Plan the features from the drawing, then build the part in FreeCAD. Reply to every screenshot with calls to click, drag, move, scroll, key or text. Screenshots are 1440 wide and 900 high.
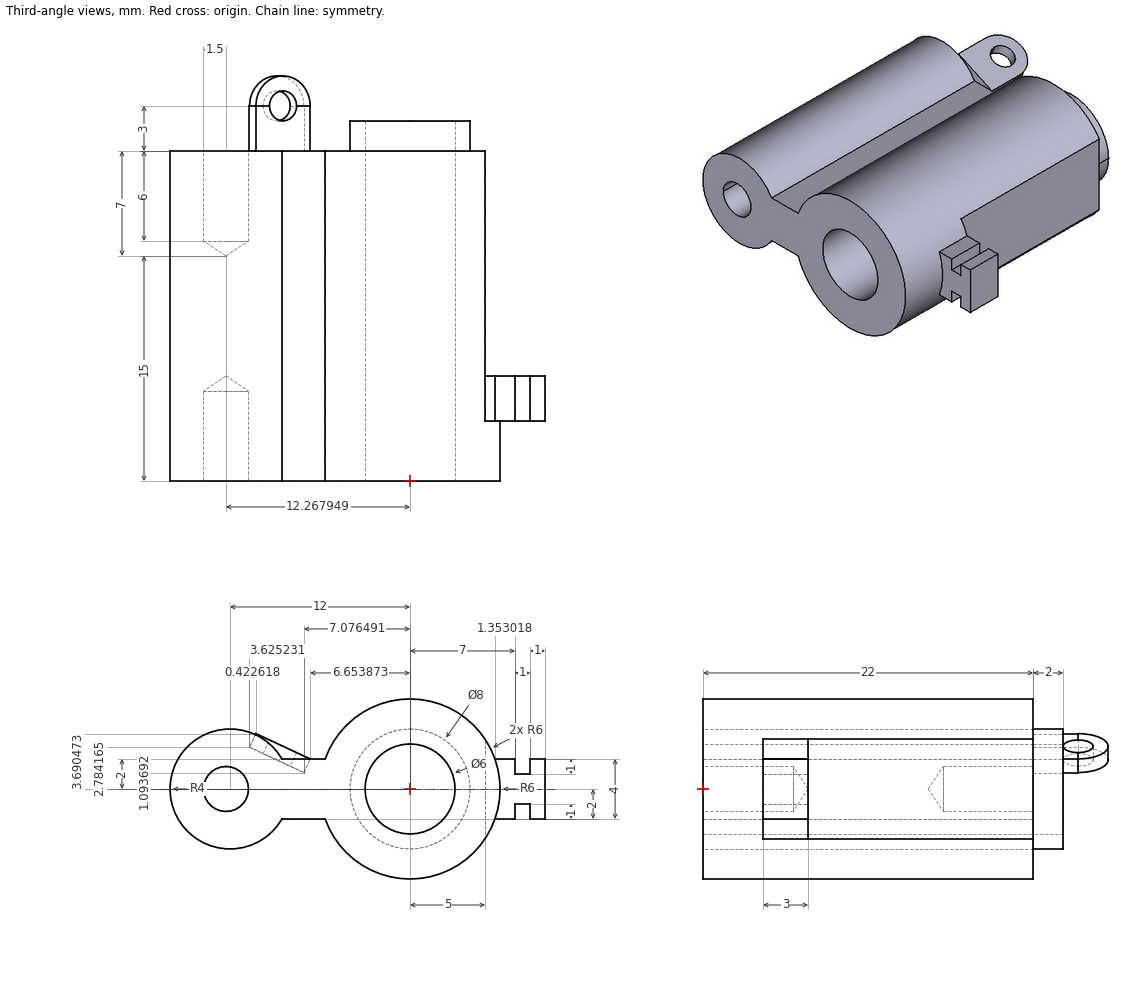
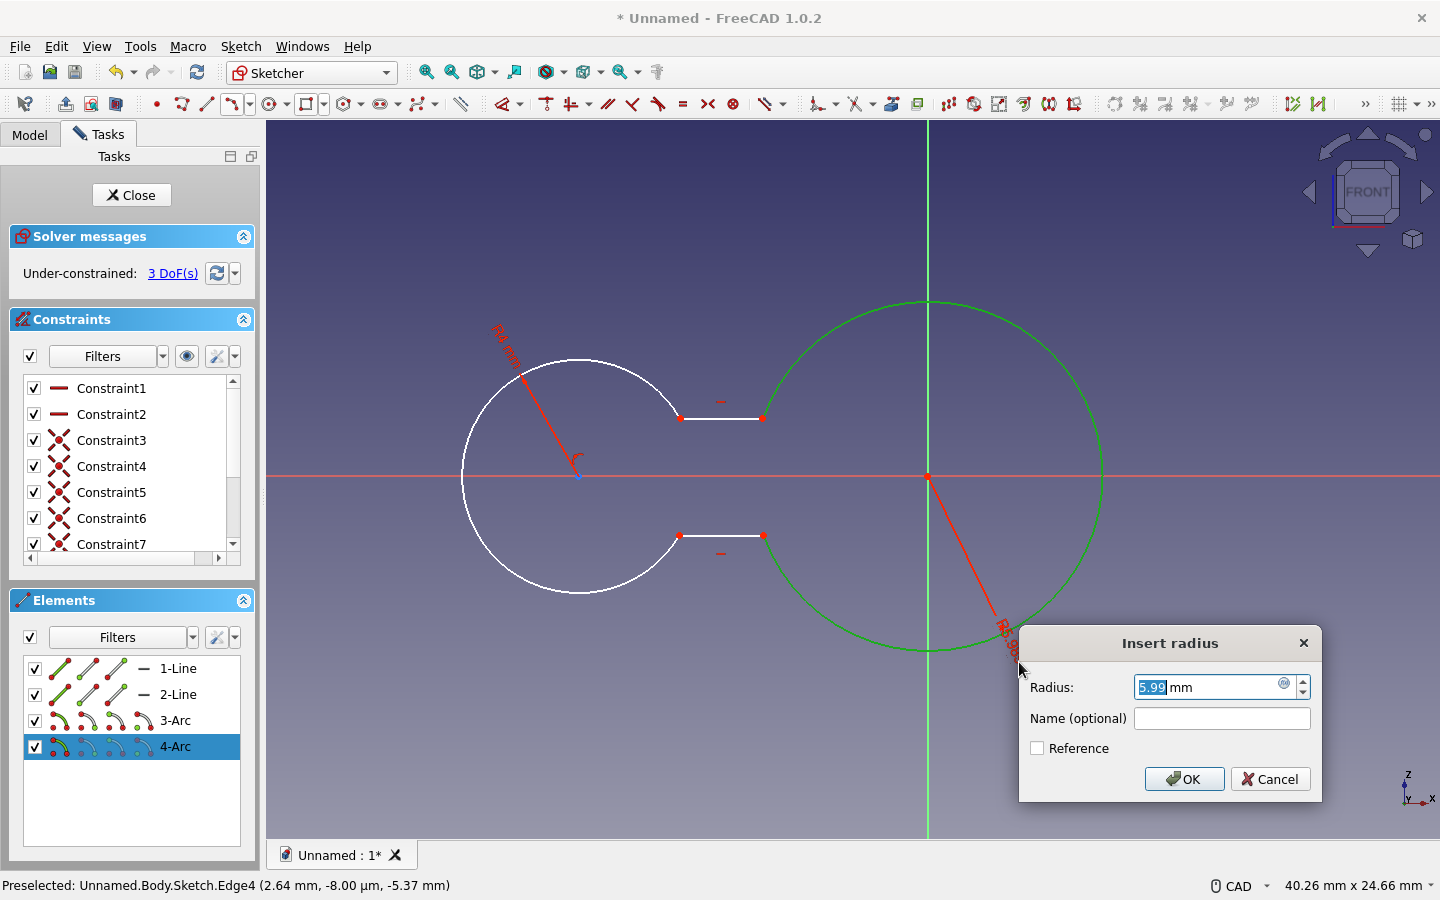
text(6)
key(Return)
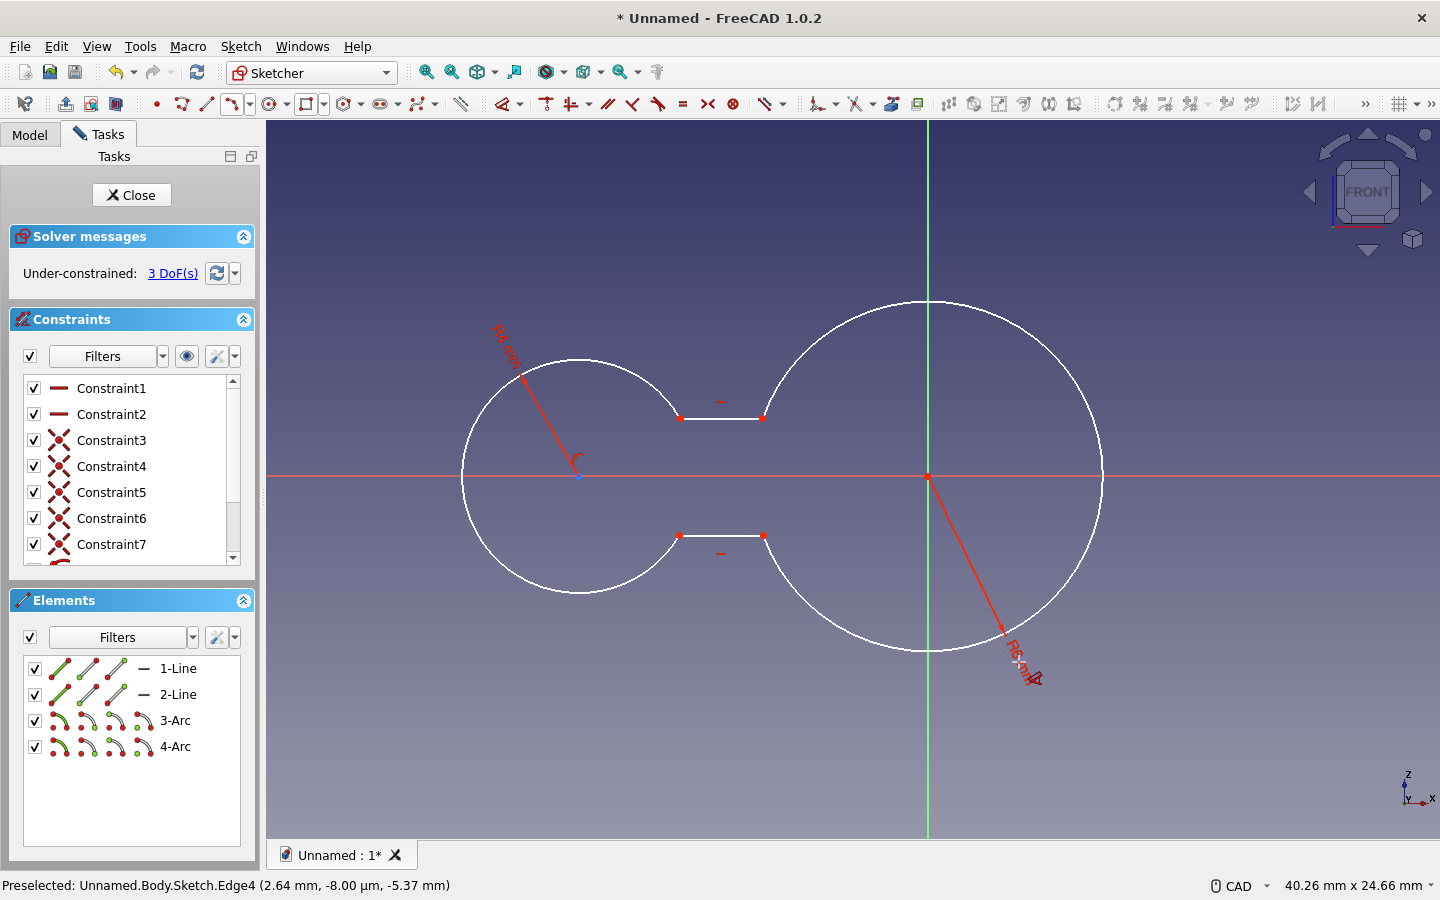
click(763, 536)
click(962, 506)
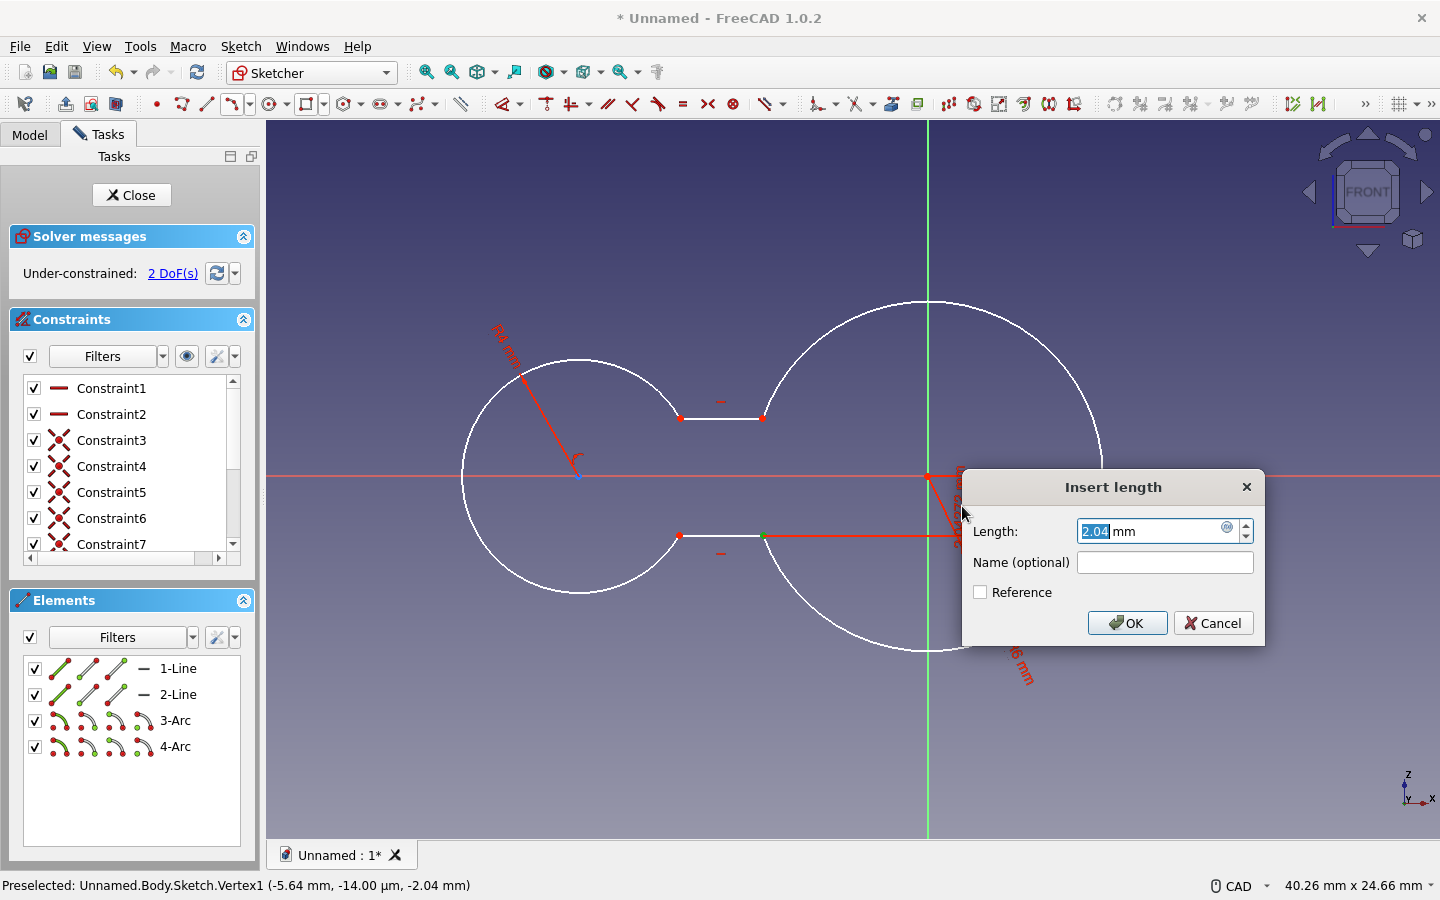
text(2)
key(Return)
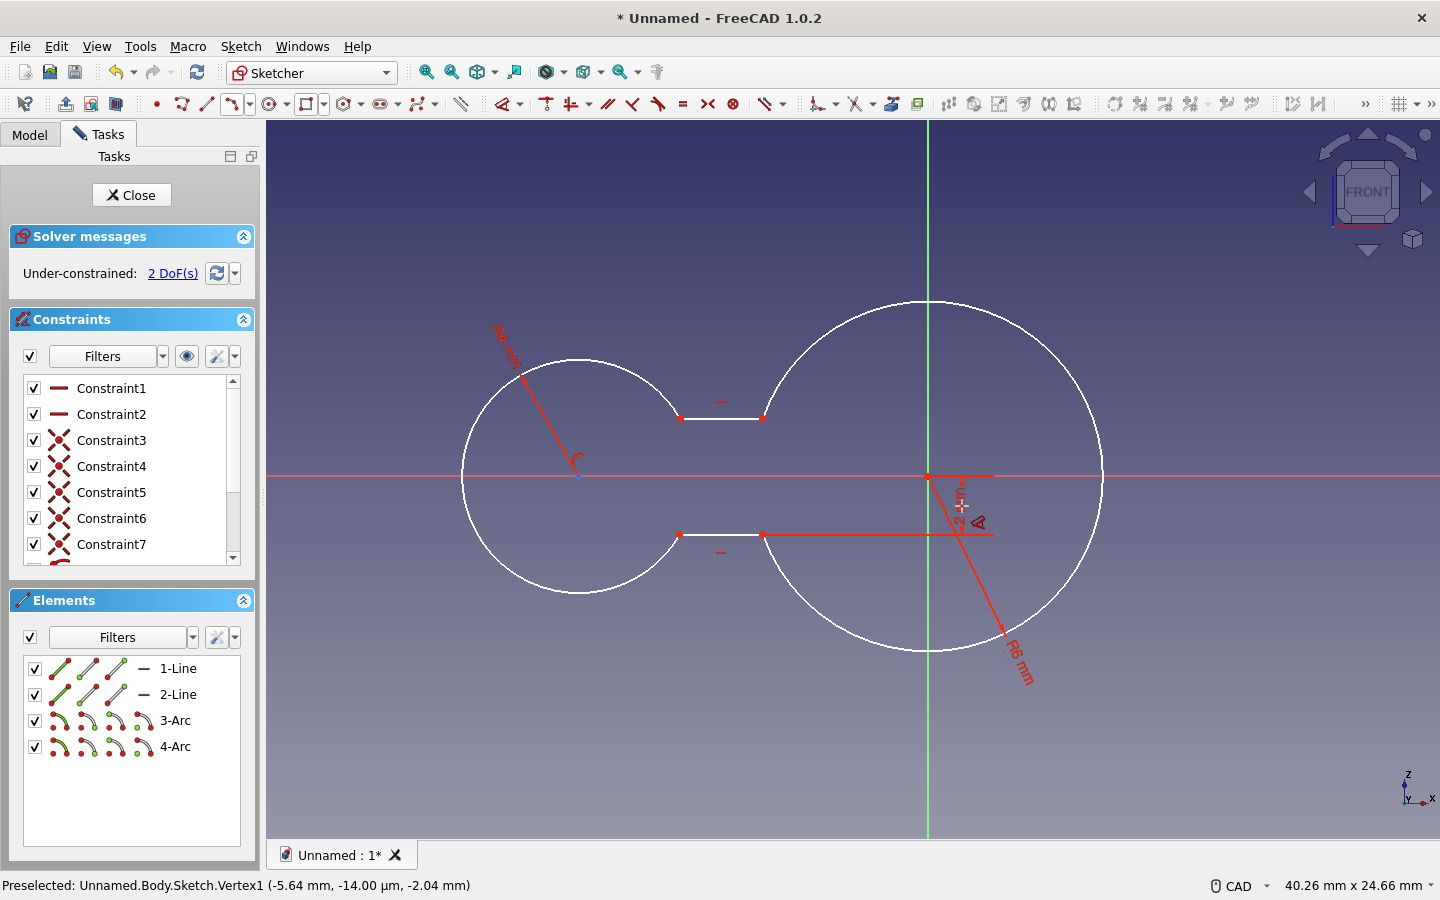
click(680, 419)
click(962, 448)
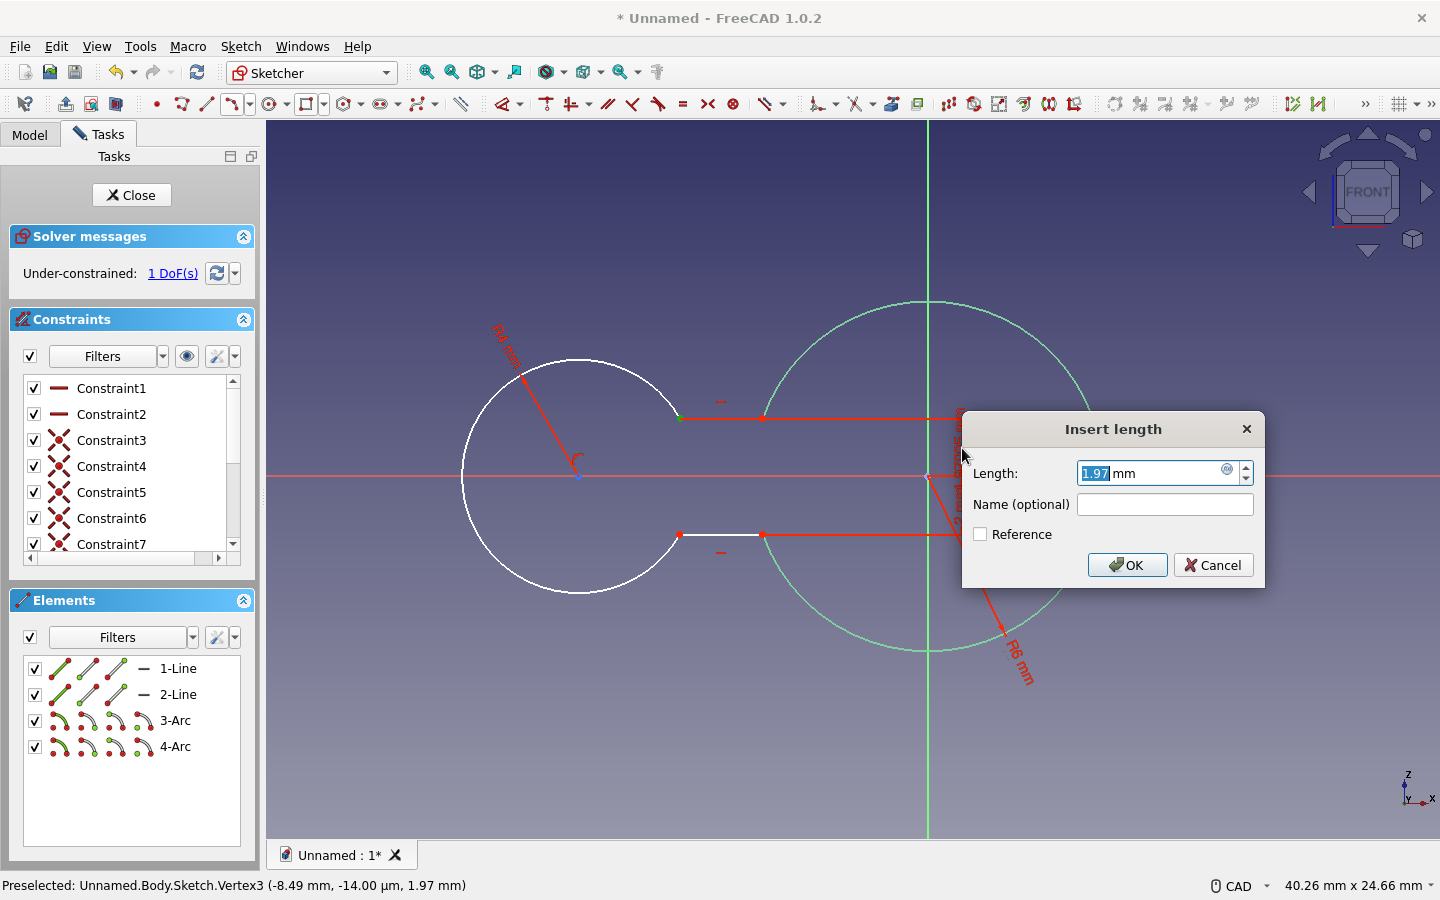
text(2)
key(Return)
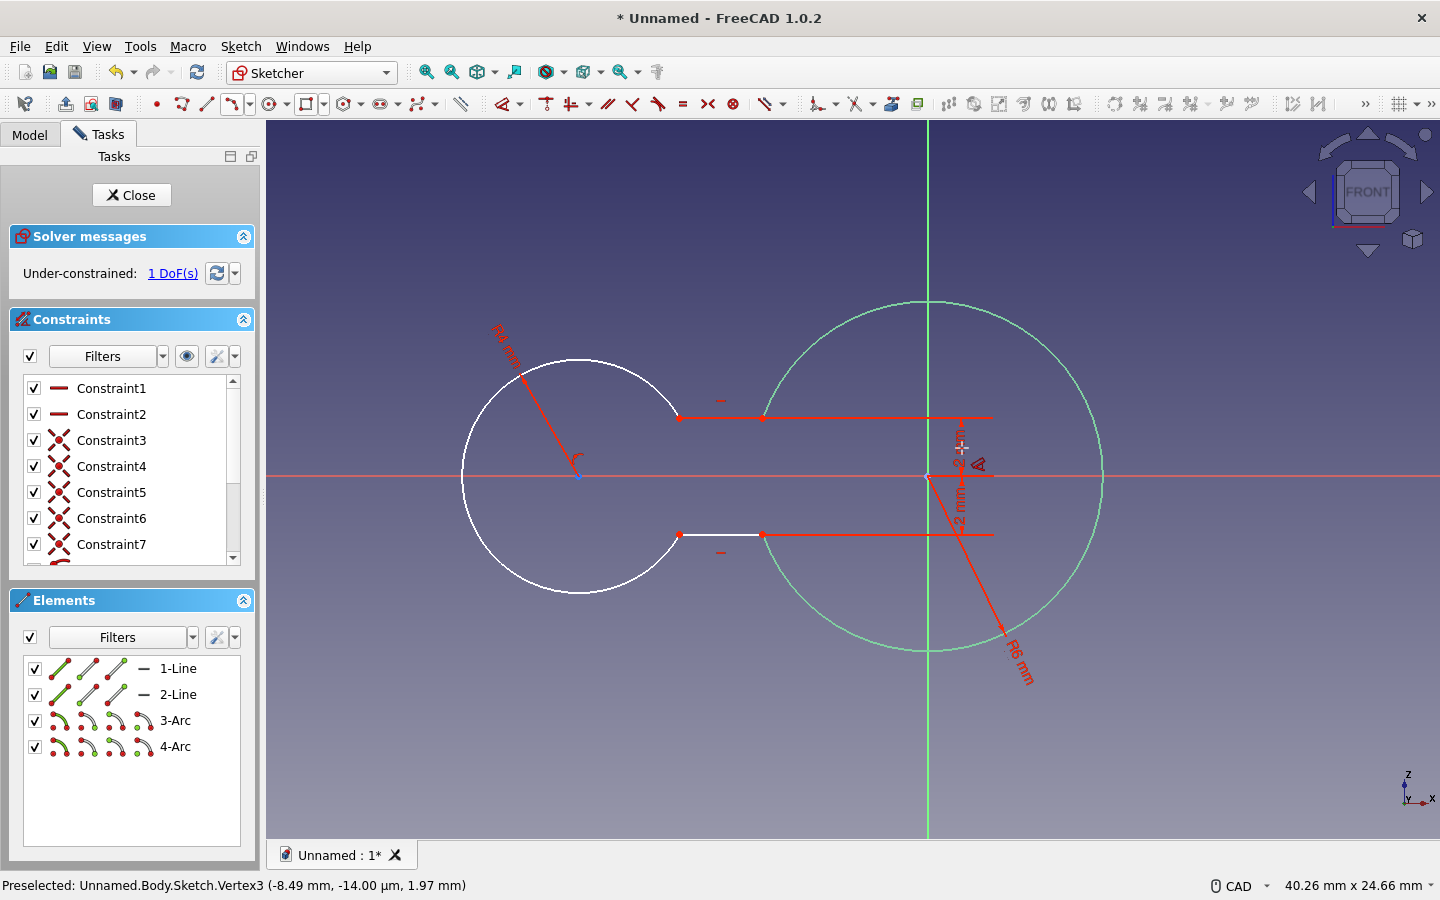
click(579, 476)
click(753, 510)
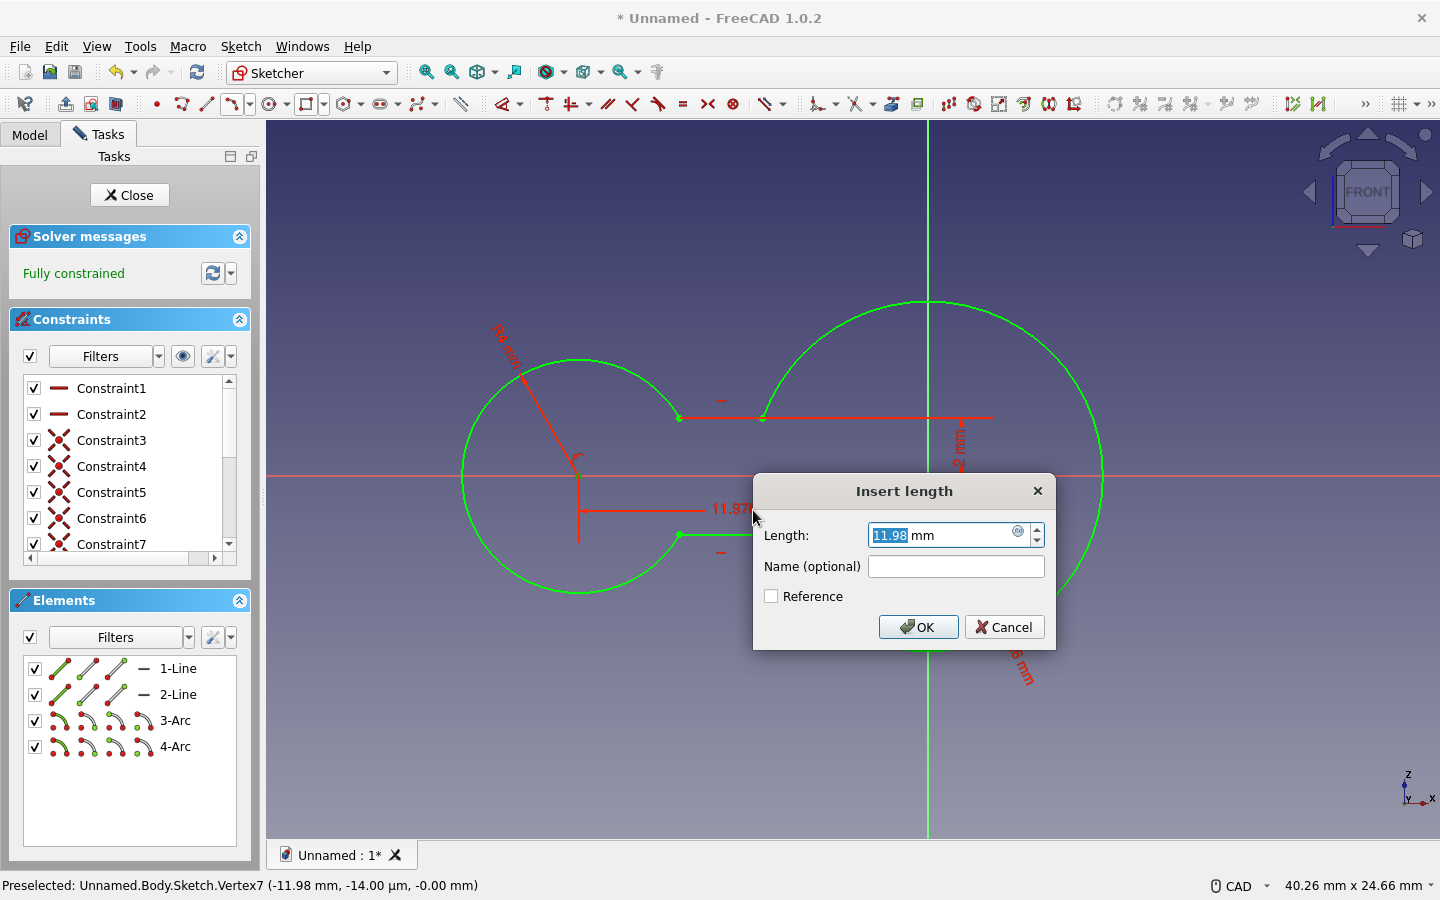
text(12)
key(Return)
key(Escape)